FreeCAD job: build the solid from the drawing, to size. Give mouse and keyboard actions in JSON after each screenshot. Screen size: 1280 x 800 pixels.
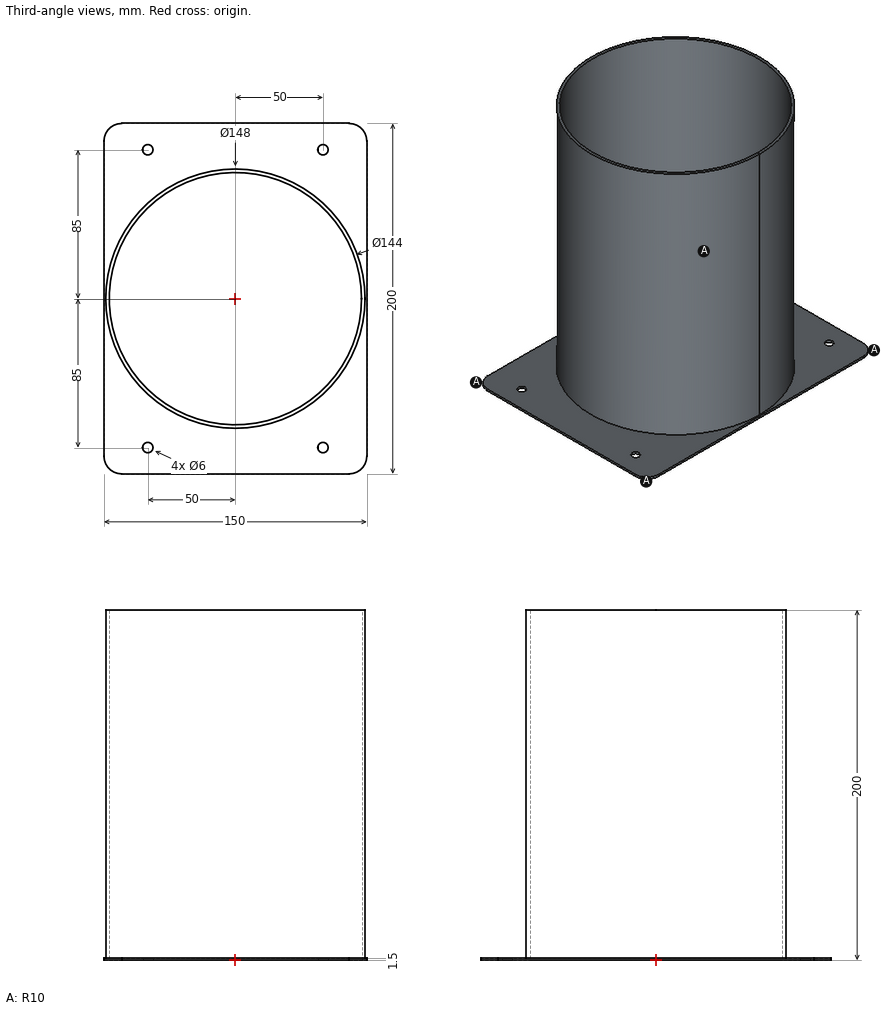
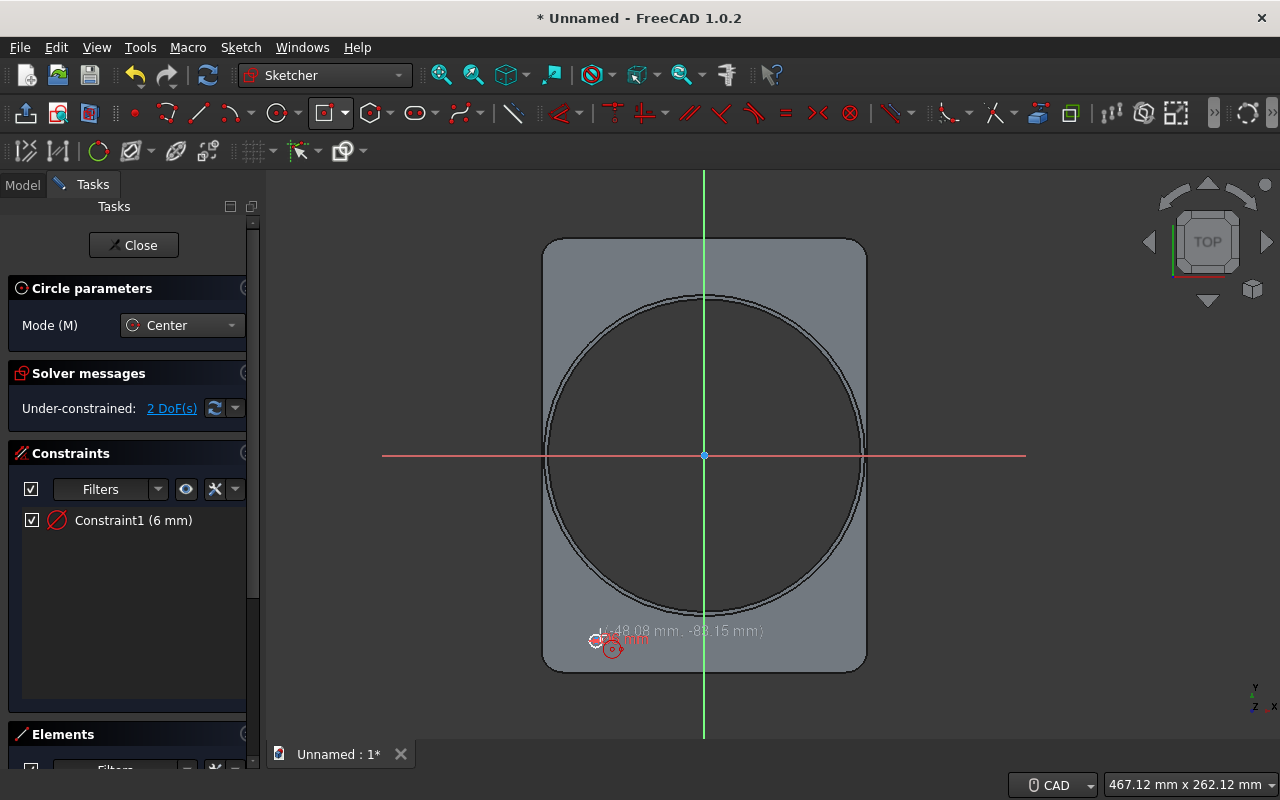
{"action": "scroll", "coordinate": [596, 271], "scroll_direction": "up", "scroll_amount": 7}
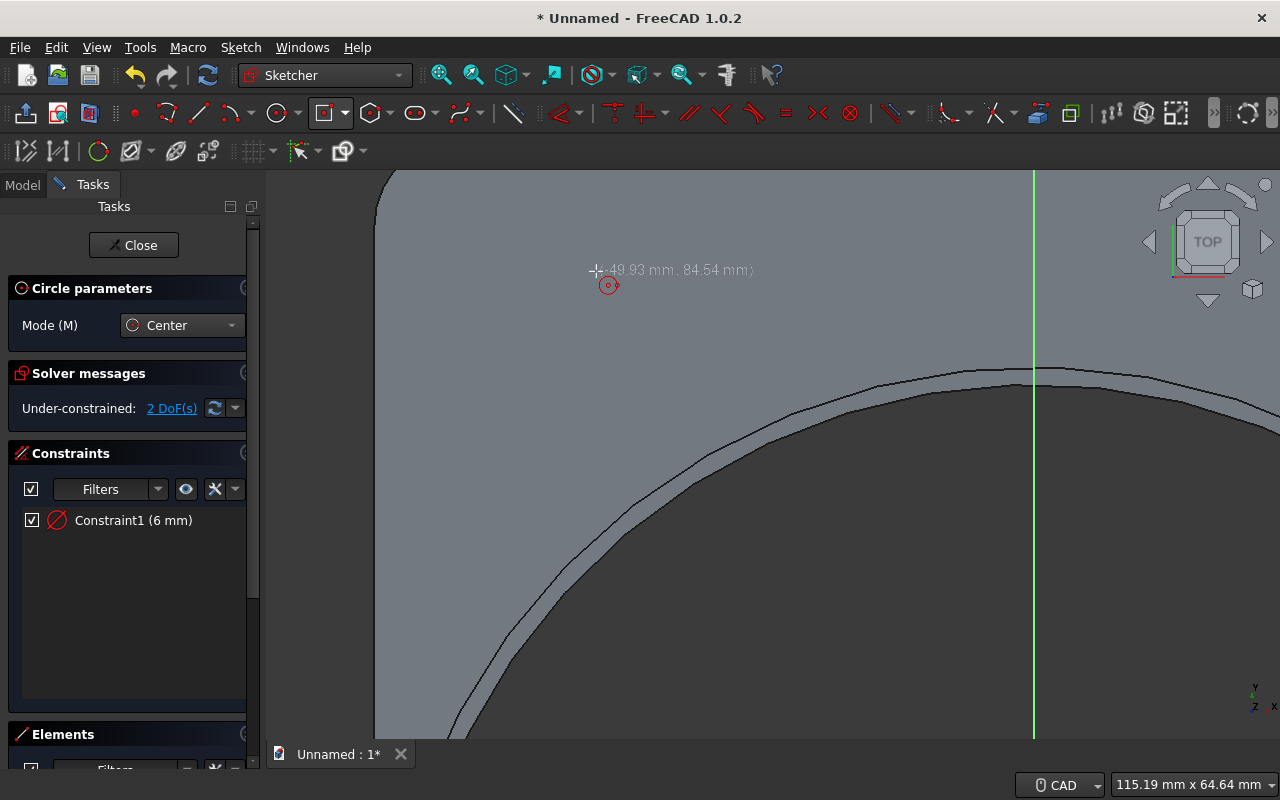
{"action": "scroll", "coordinate": [596, 270], "scroll_direction": "down", "scroll_amount": 7}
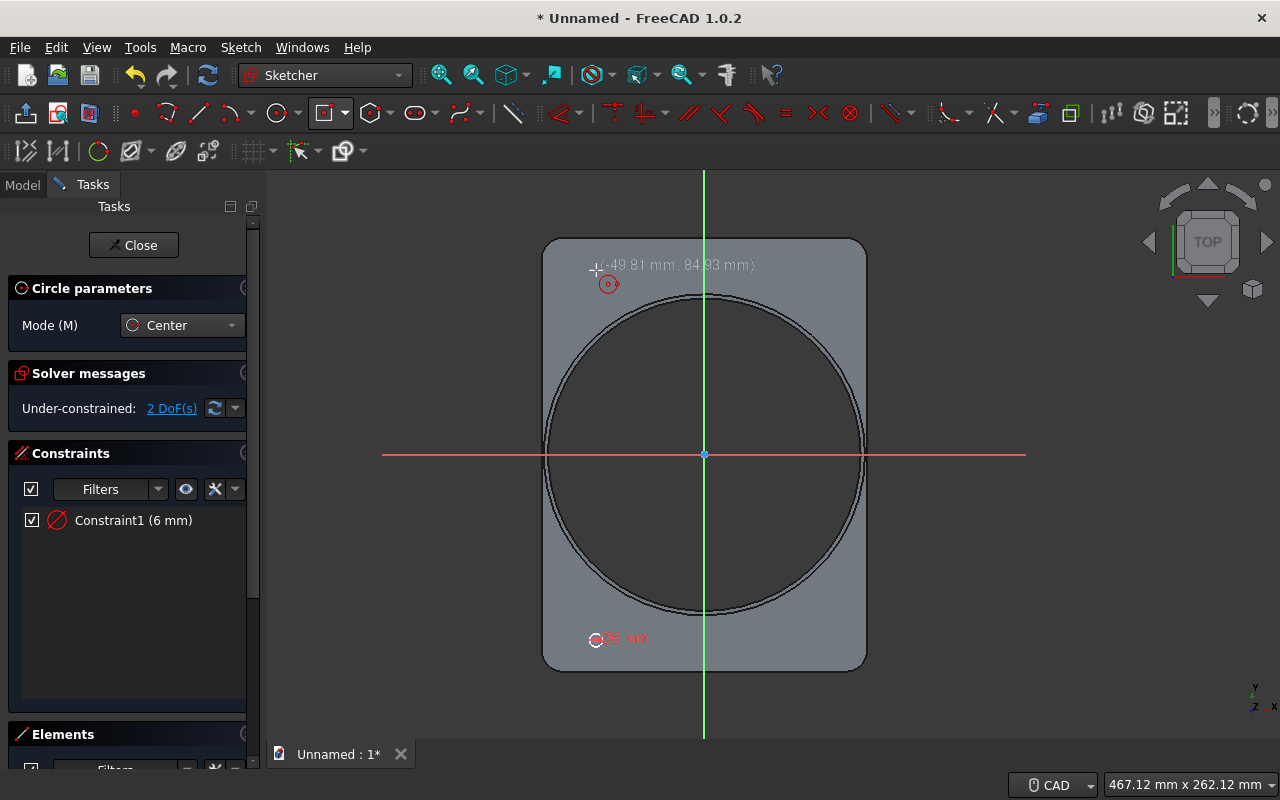
{"action": "left_click", "coordinate": [596, 270]}
{"action": "mouse_move", "coordinate": [600, 266]}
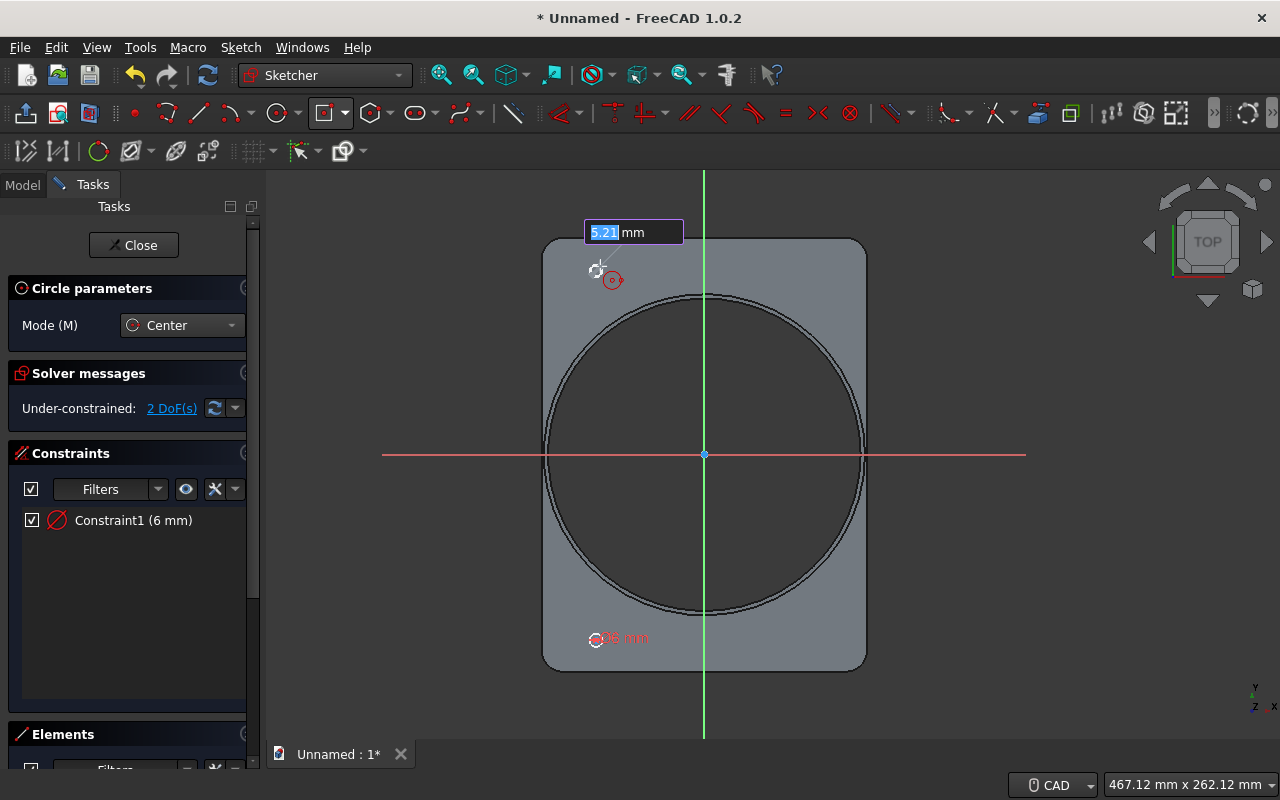
{"action": "type", "text": "6"}
{"action": "key", "text": "Return"}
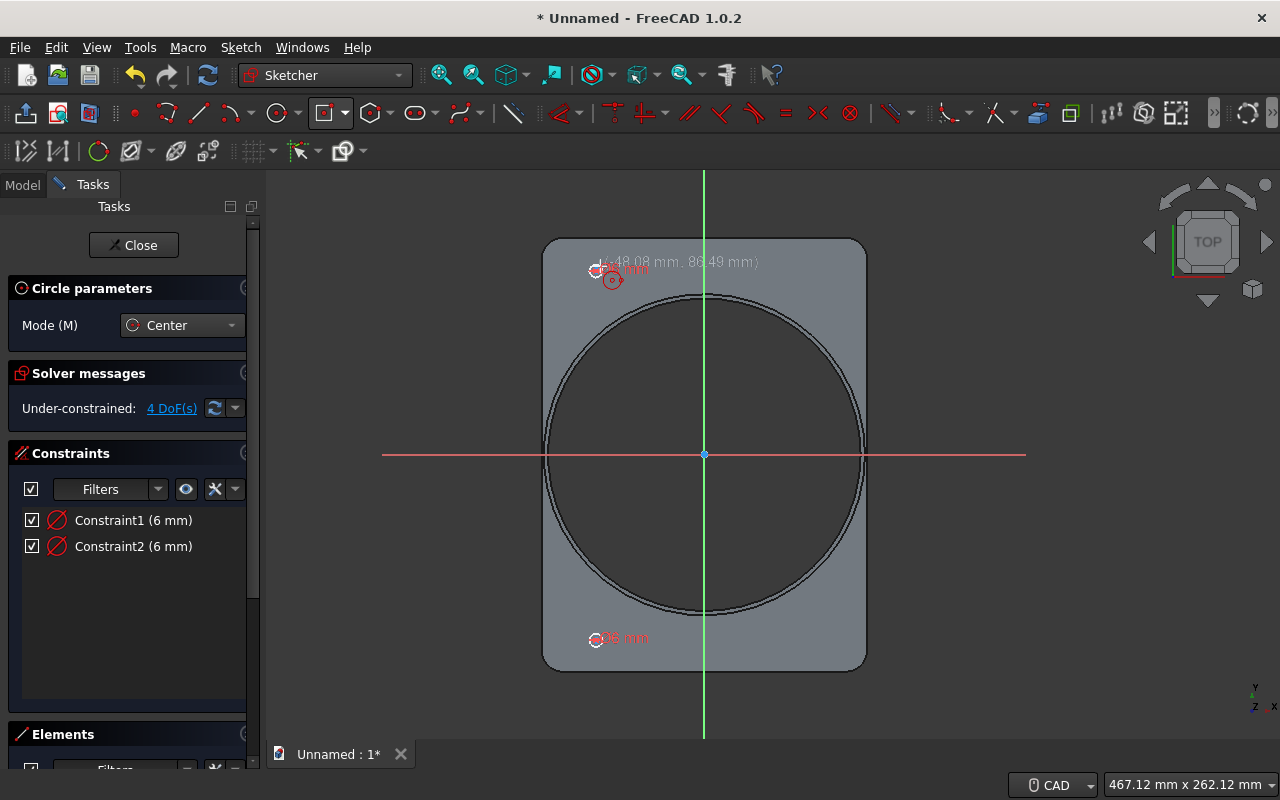
{"action": "scroll", "coordinate": [813, 270], "scroll_direction": "up", "scroll_amount": 7}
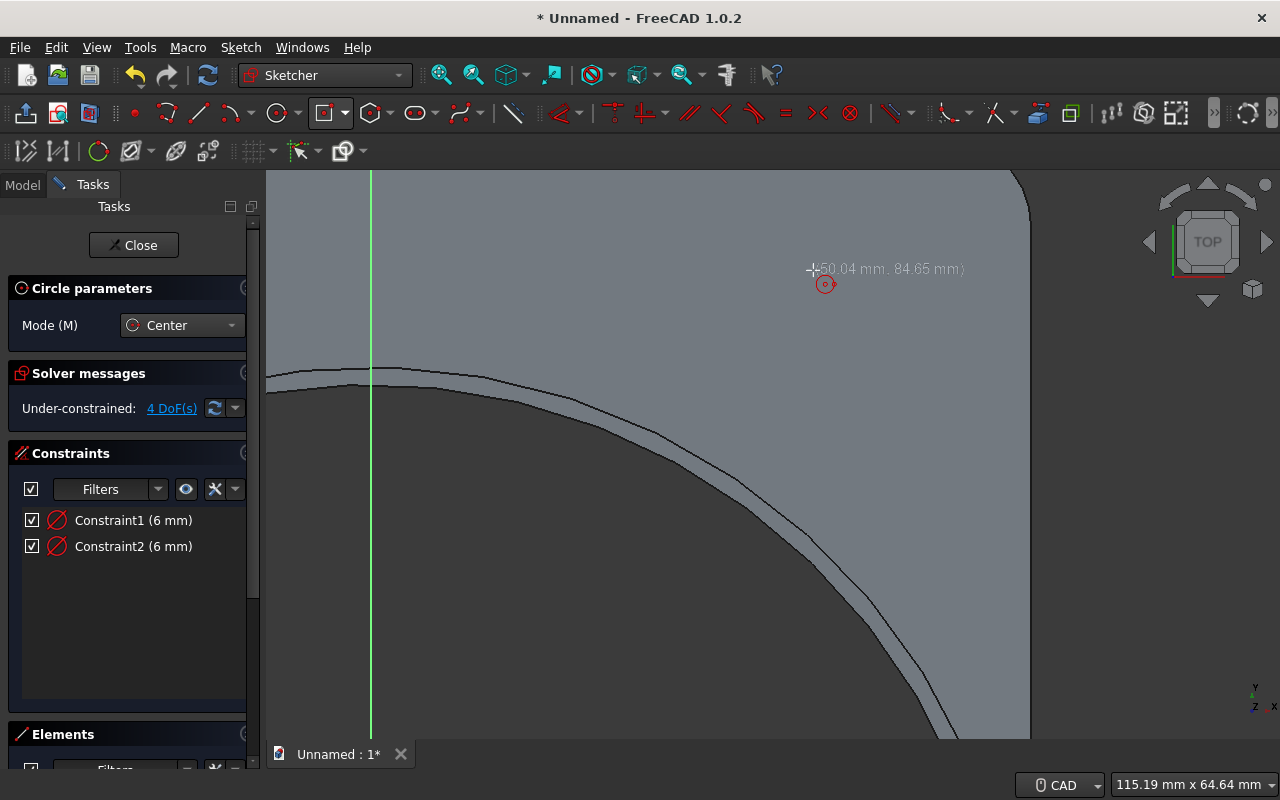
{"action": "scroll", "coordinate": [814, 270], "scroll_direction": "down", "scroll_amount": 7}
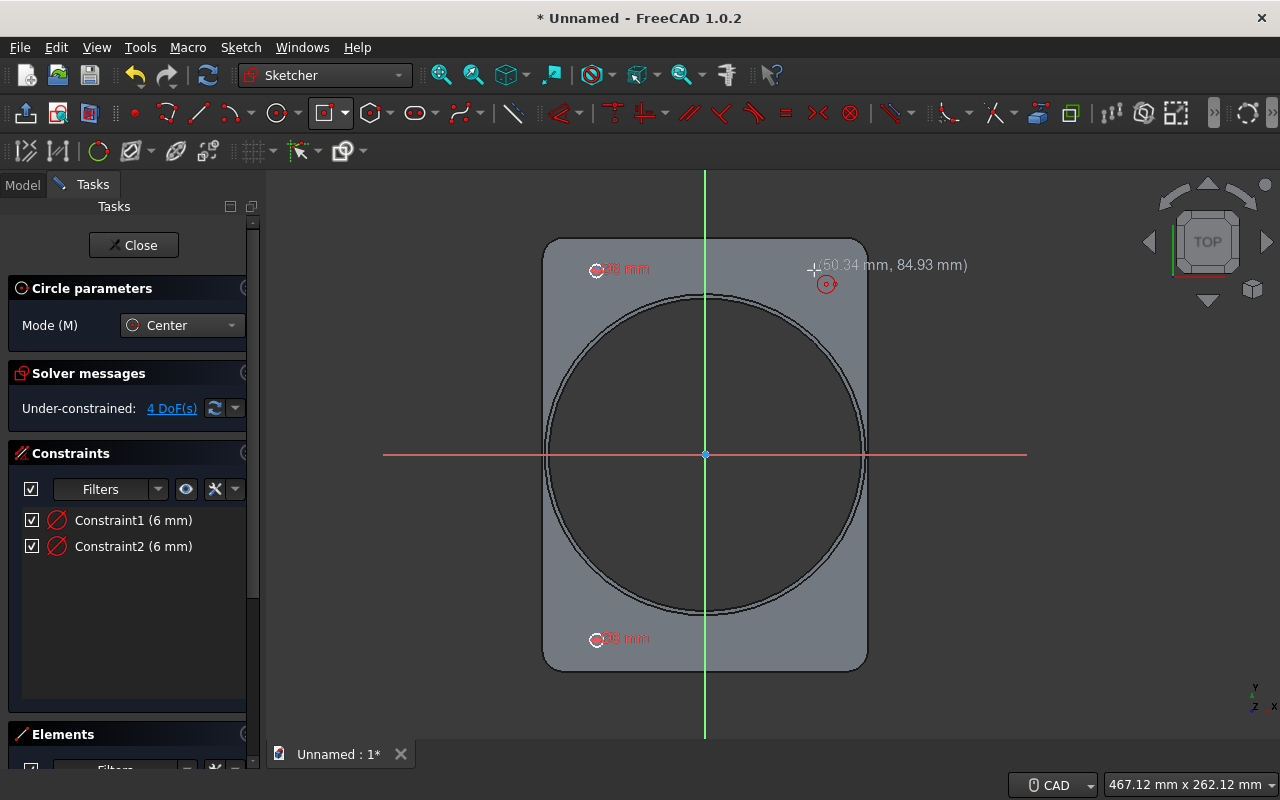
{"action": "left_click", "coordinate": [814, 270]}
{"action": "mouse_move", "coordinate": [818, 266]}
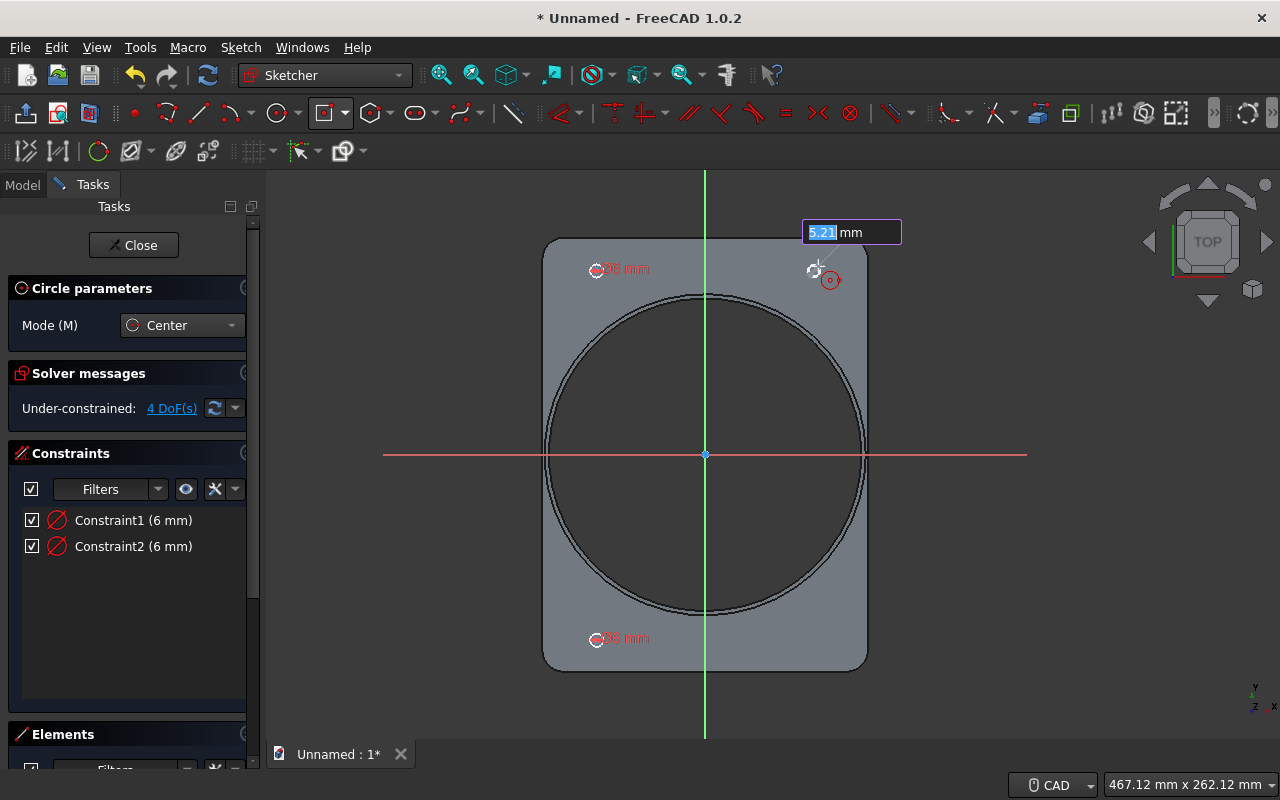
{"action": "type", "text": "6"}
{"action": "key", "text": "Return"}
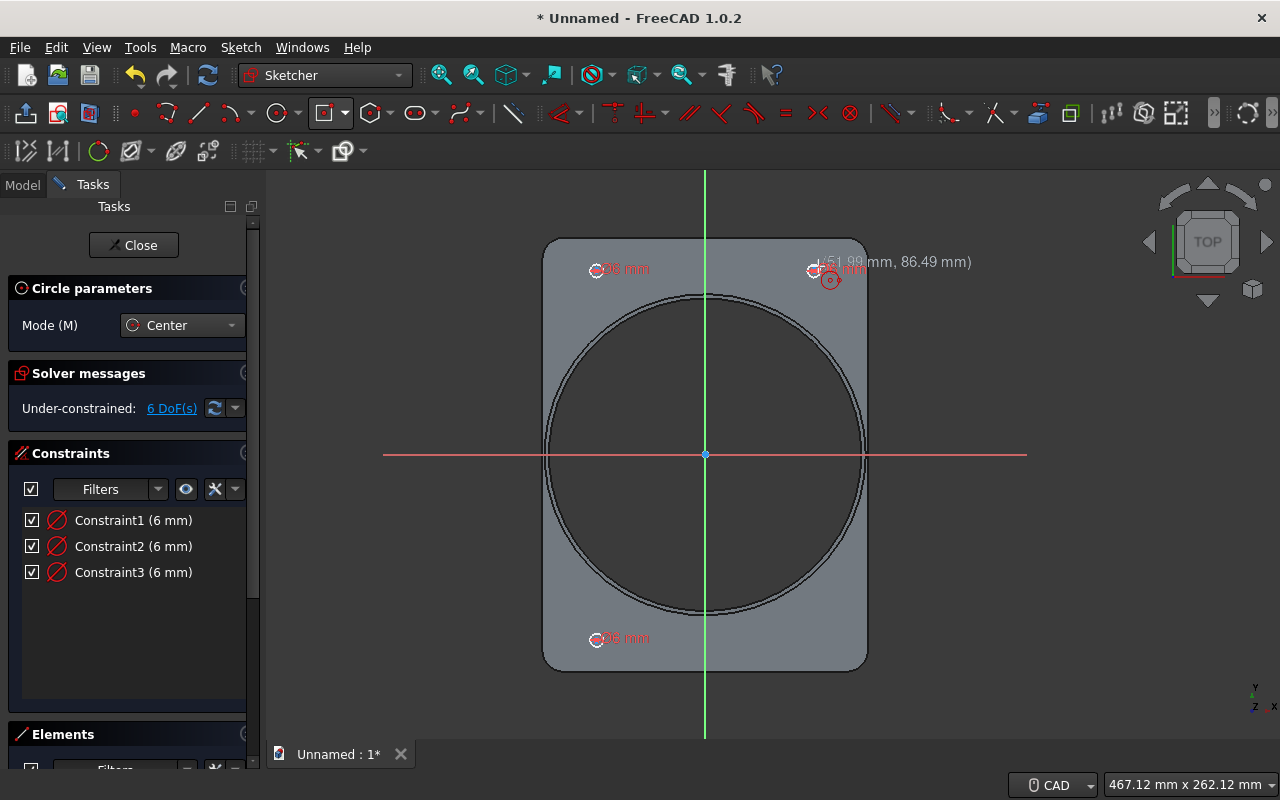
{"action": "scroll", "coordinate": [814, 639], "scroll_direction": "up", "scroll_amount": 7}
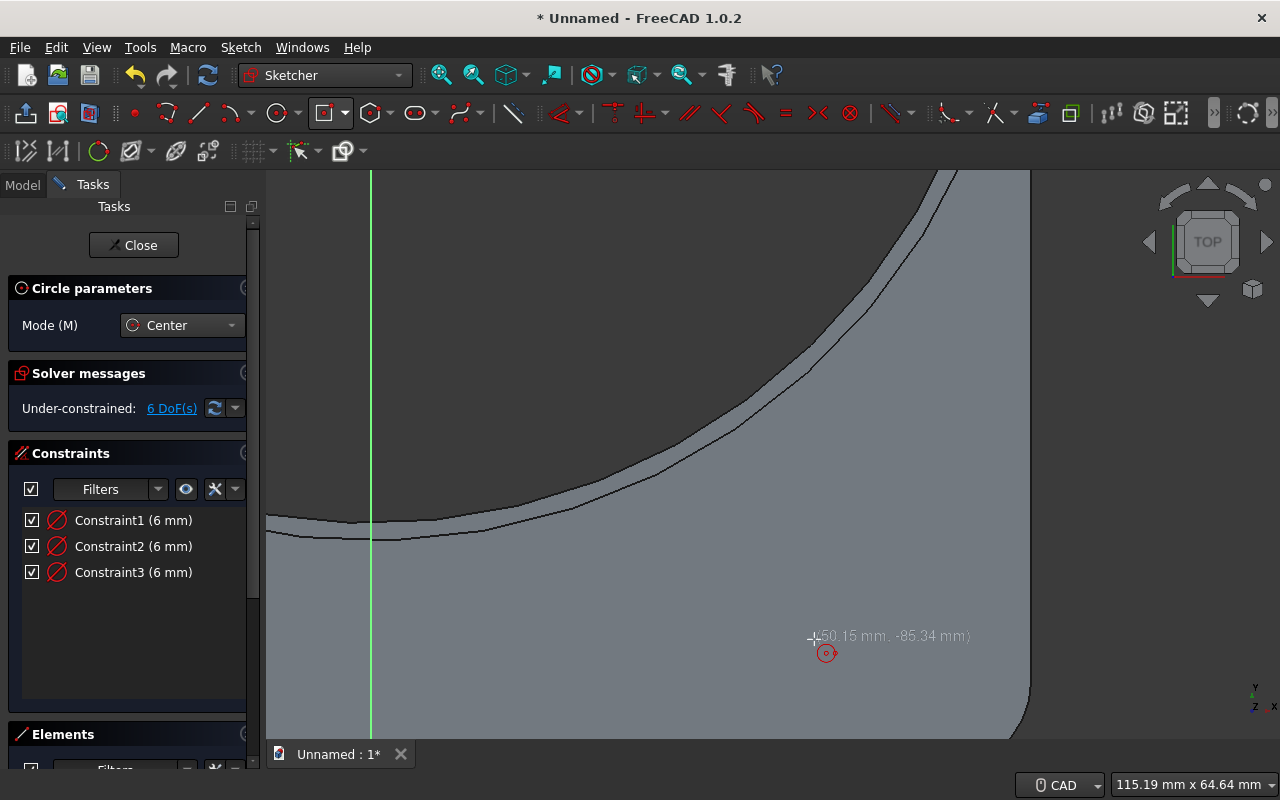
{"action": "scroll", "coordinate": [814, 639], "scroll_direction": "down", "scroll_amount": 7}